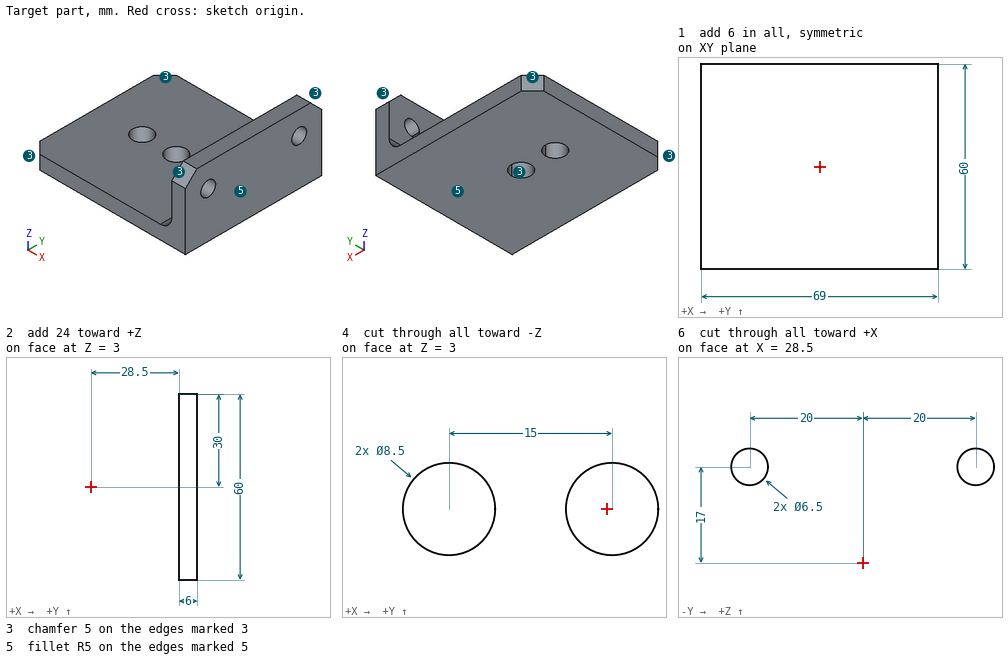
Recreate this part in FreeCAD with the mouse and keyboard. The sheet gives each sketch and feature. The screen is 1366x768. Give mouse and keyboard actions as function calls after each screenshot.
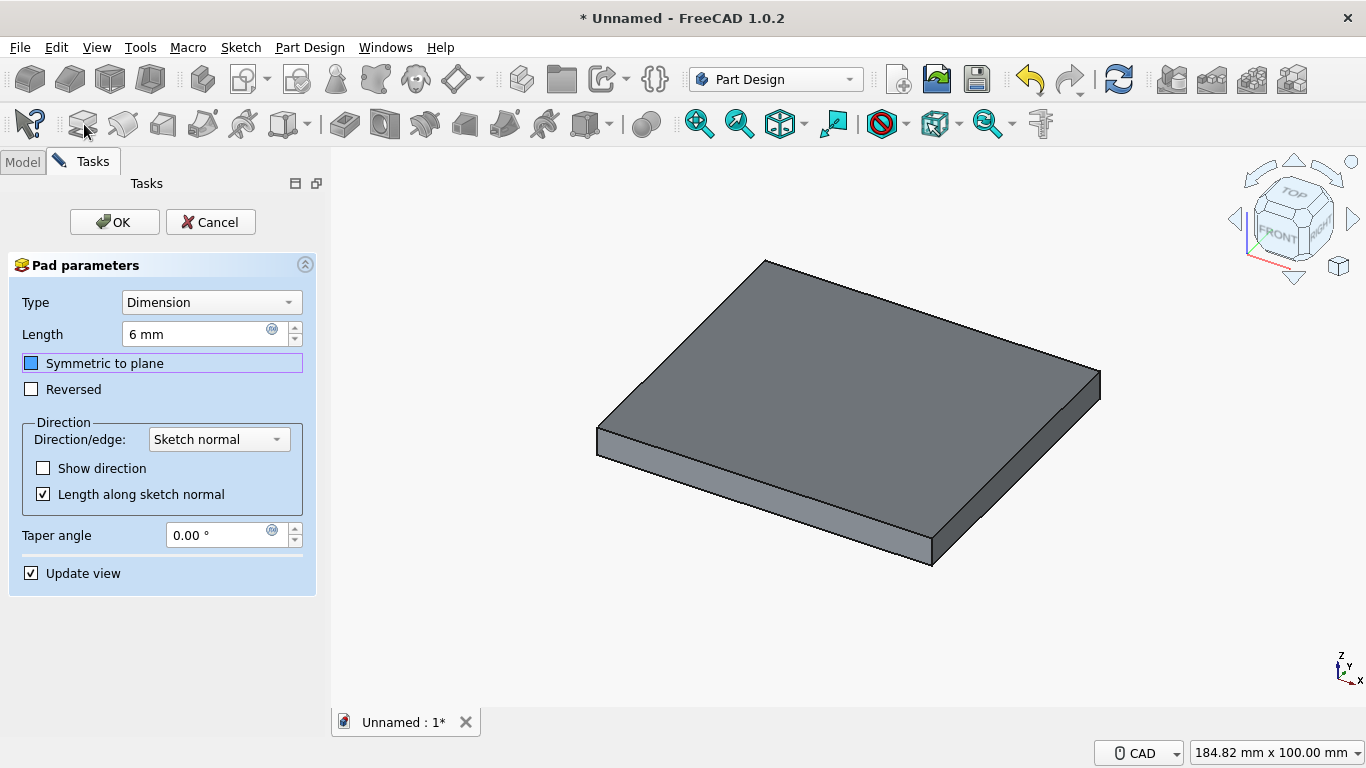
click(30, 363)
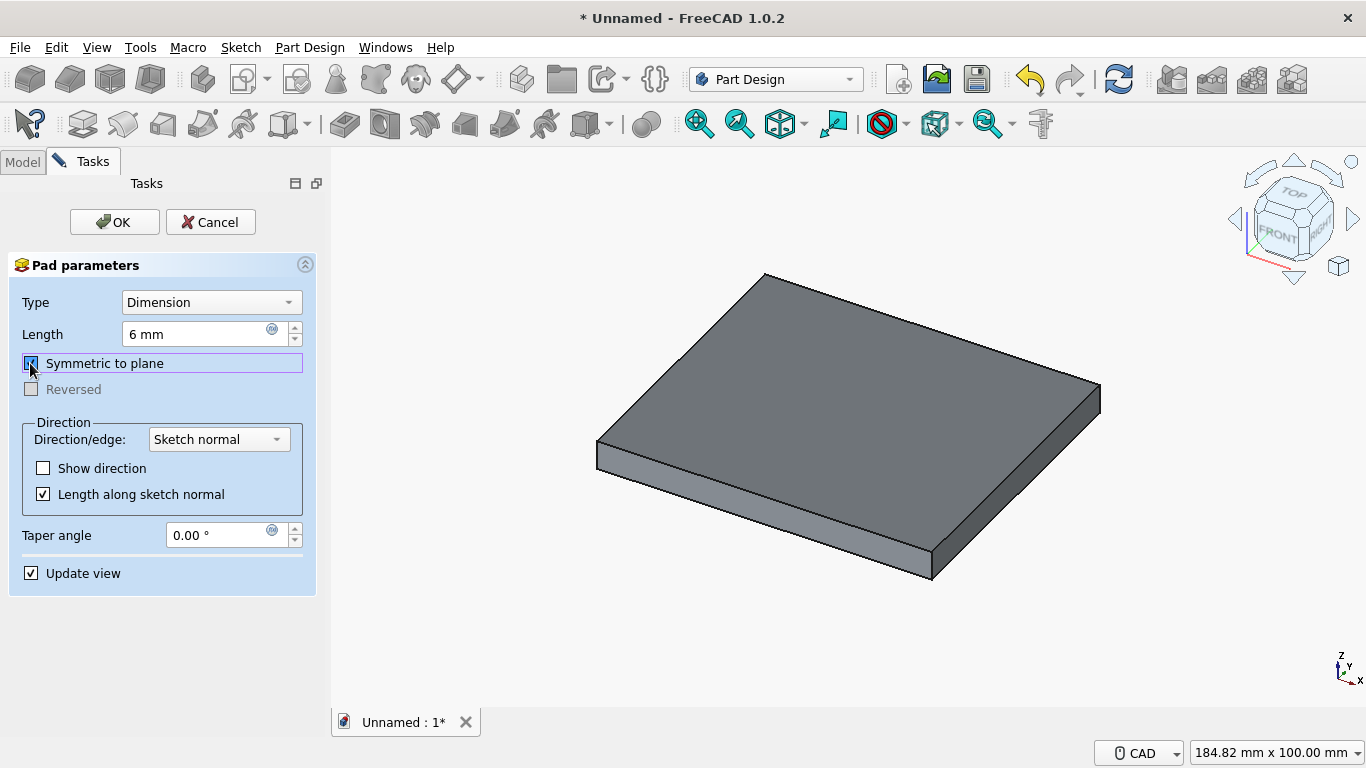
click(115, 222)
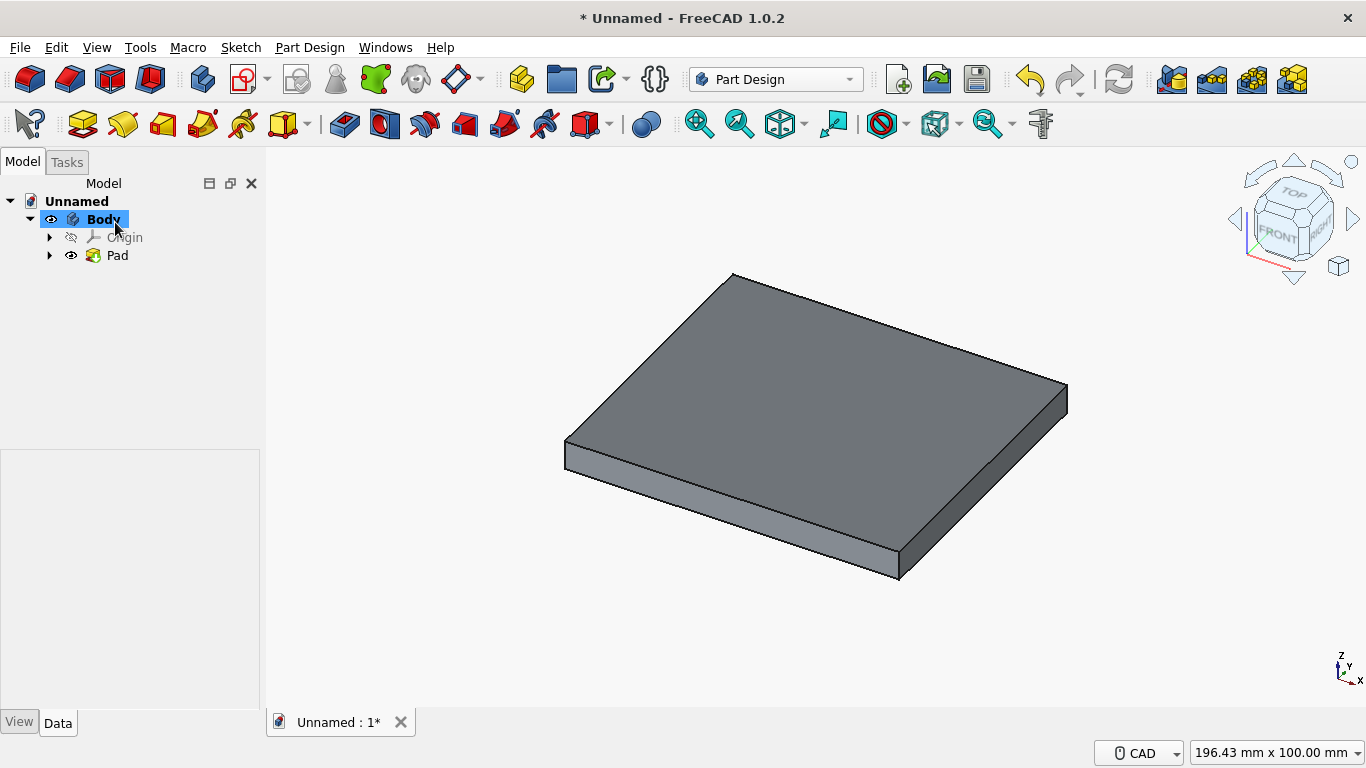
click(816, 412)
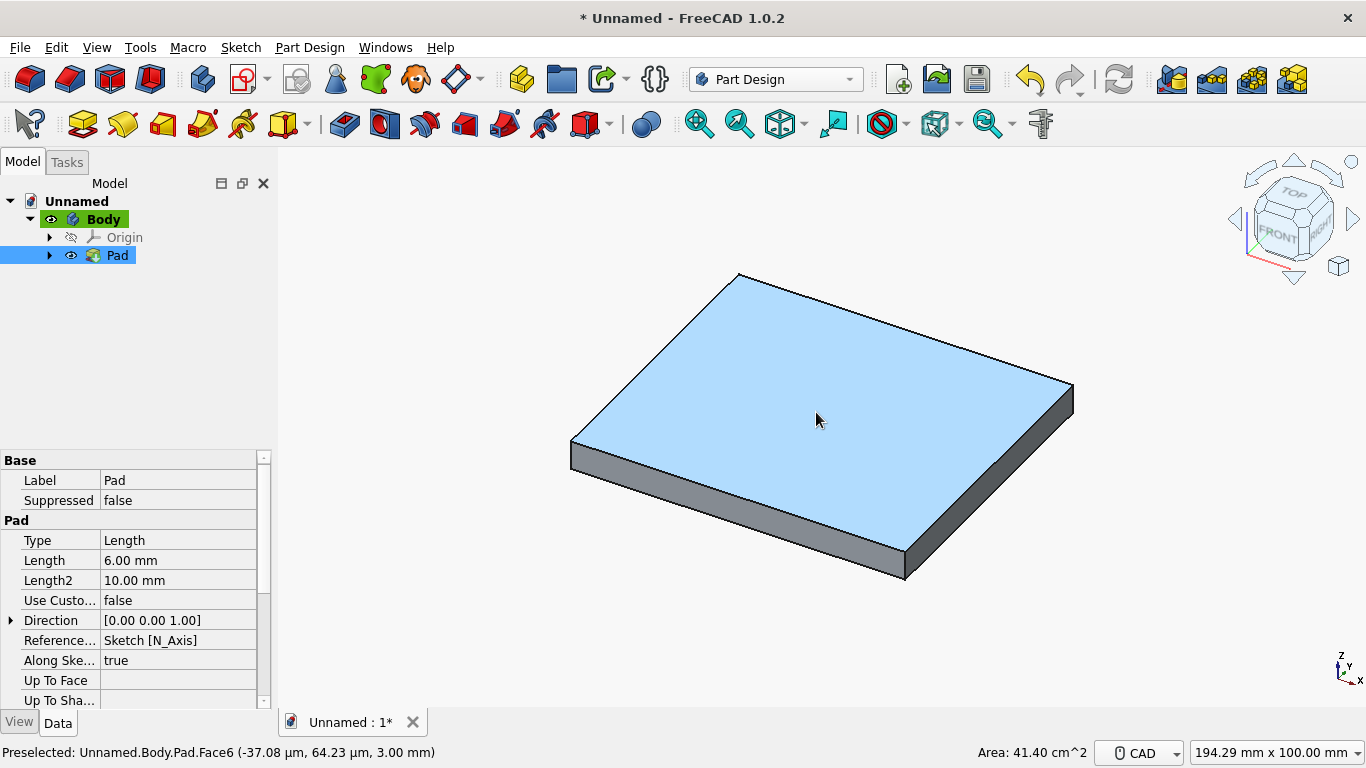
click(244, 80)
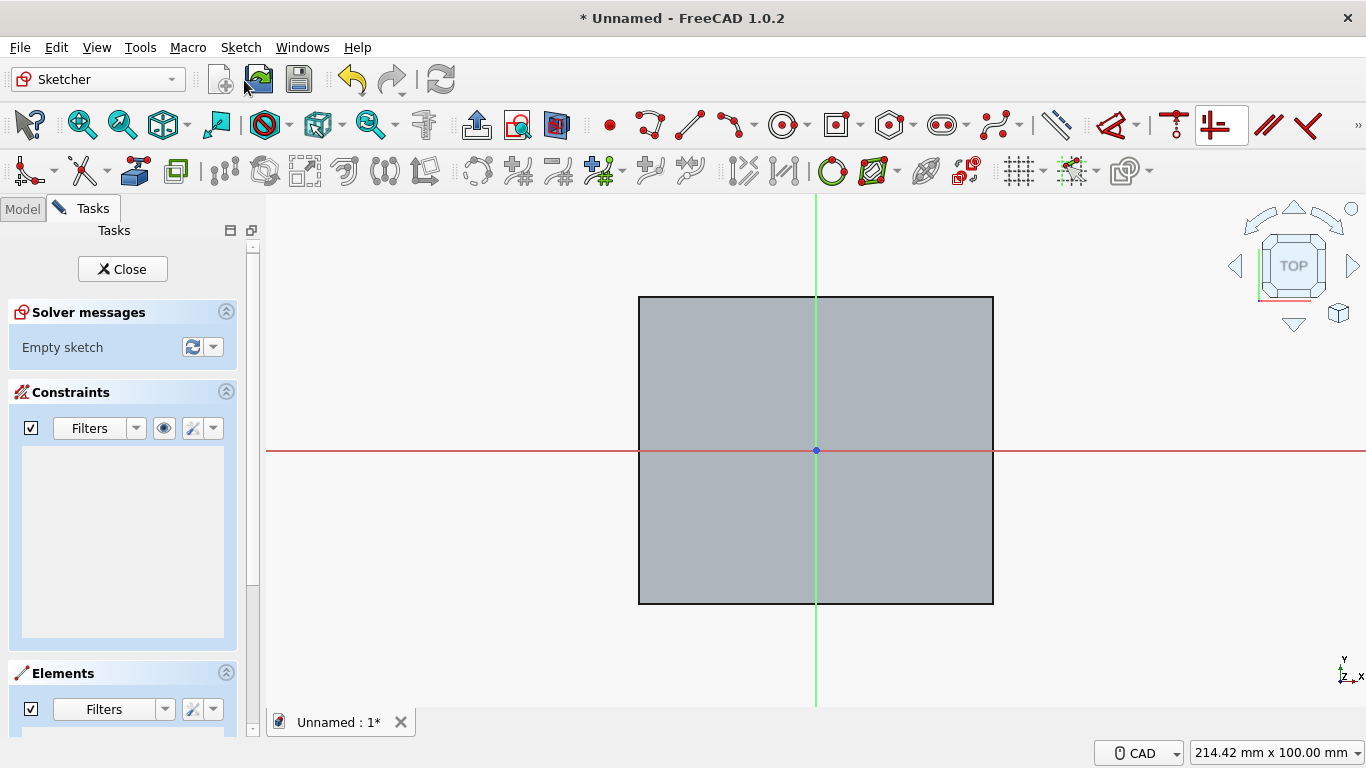
key(g)
key(r)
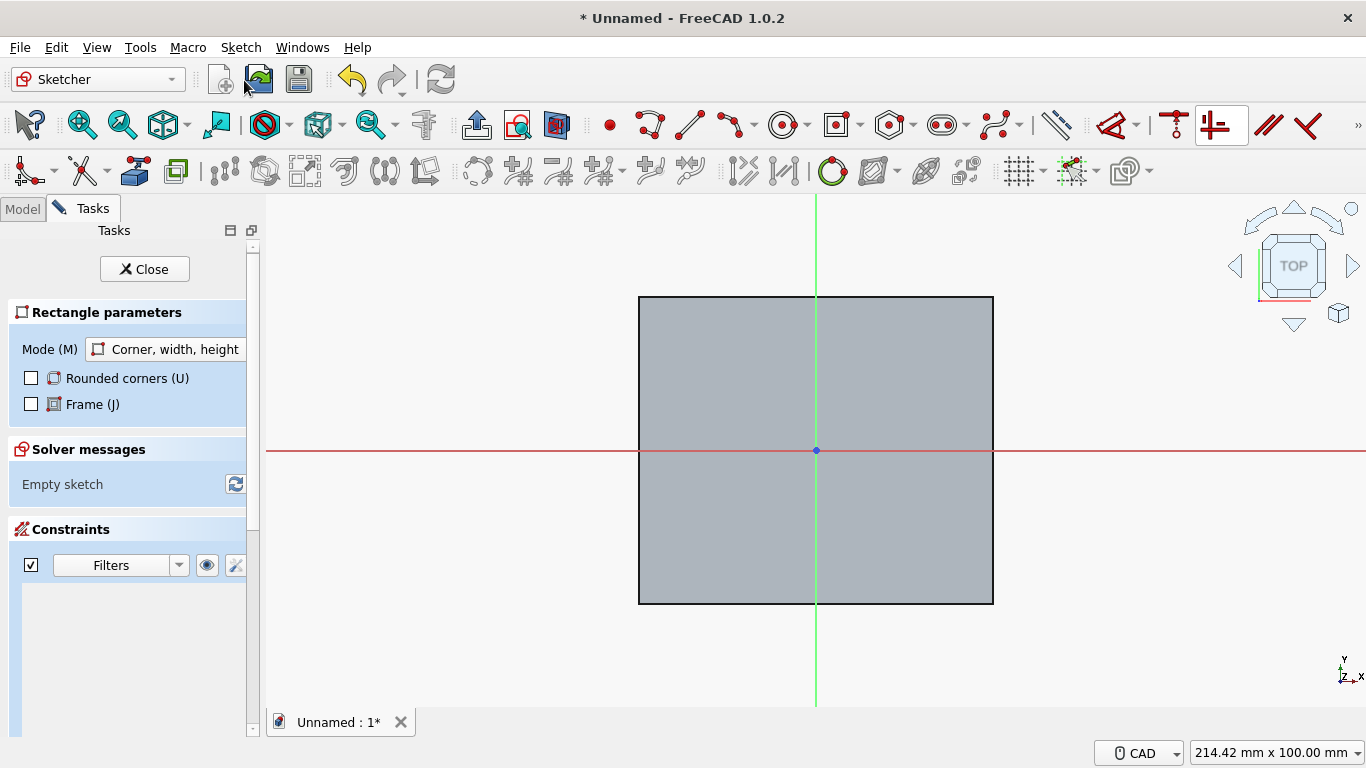
click(962, 297)
move(993, 604)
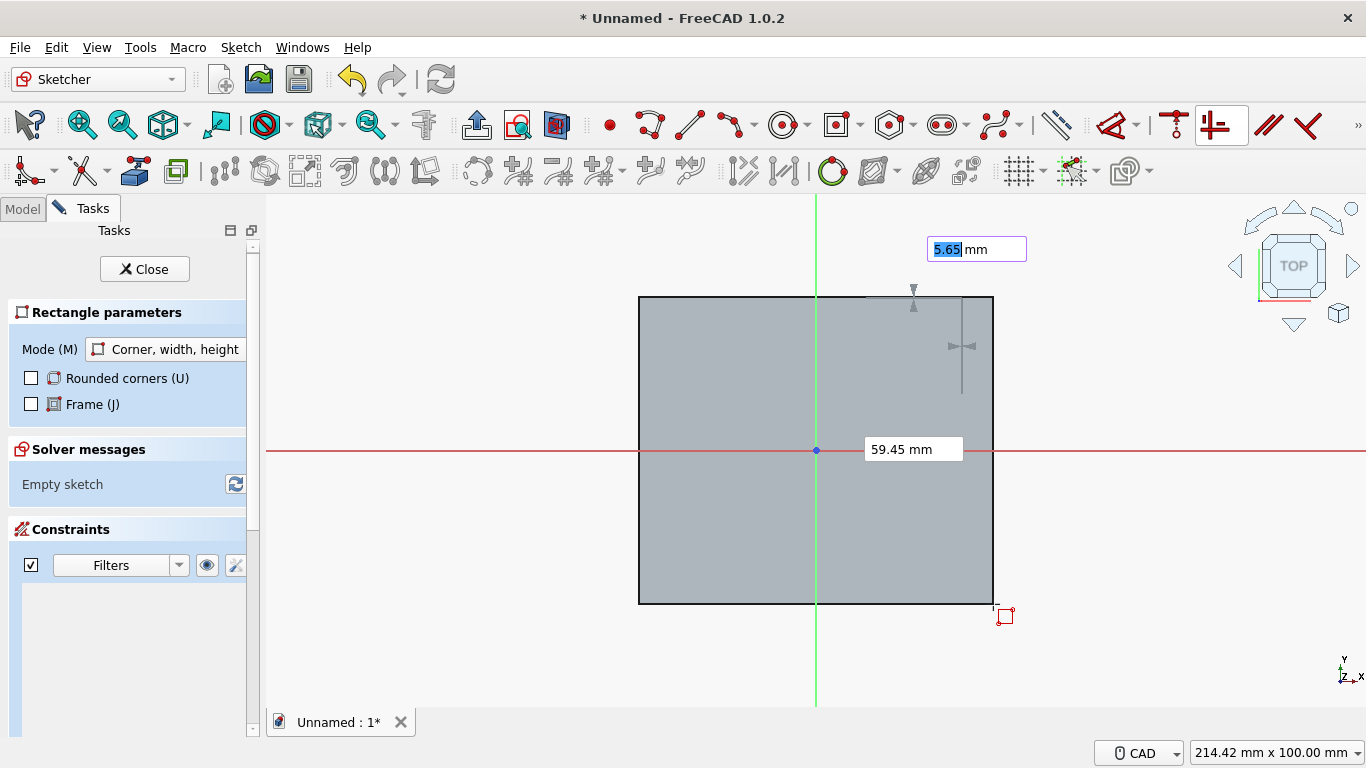
text(6)
key(Tab)
text(60)
key(Return)
key(Escape)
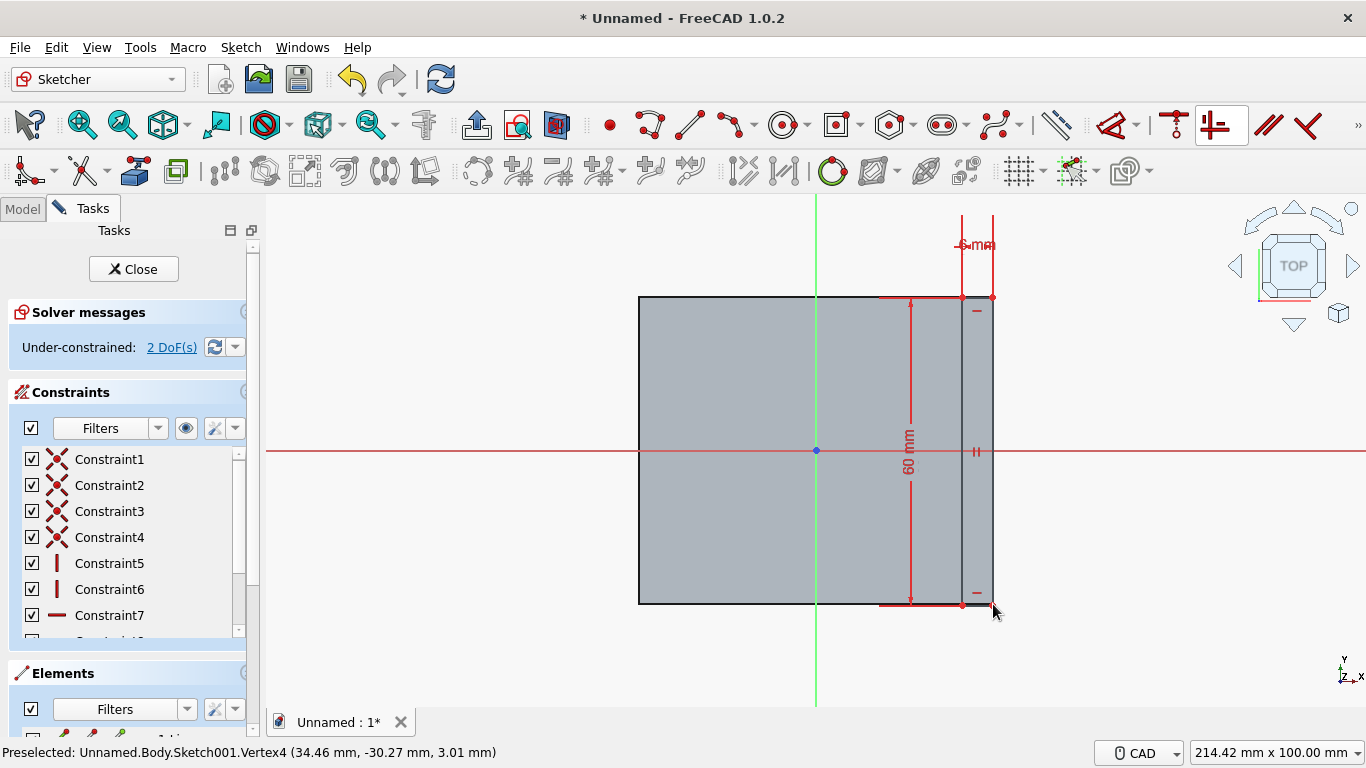
click(962, 298)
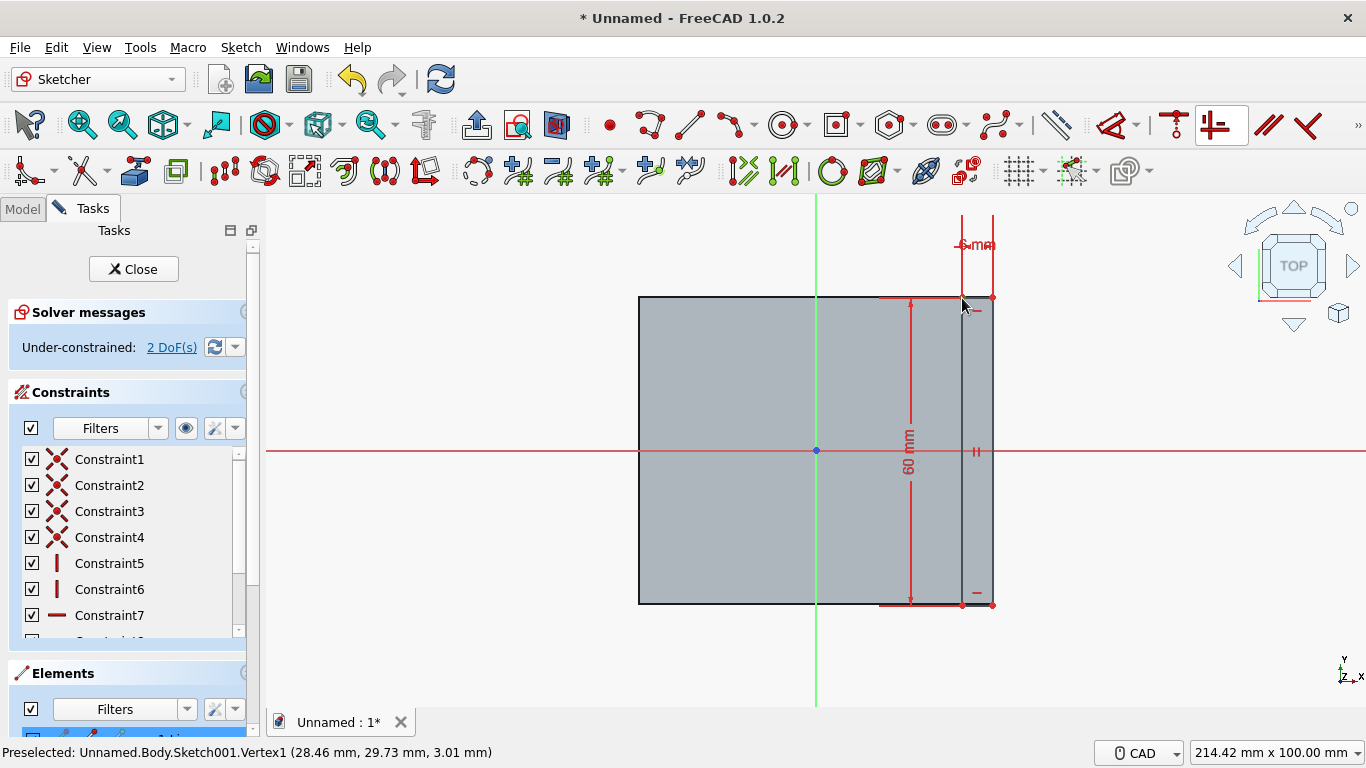
key(i)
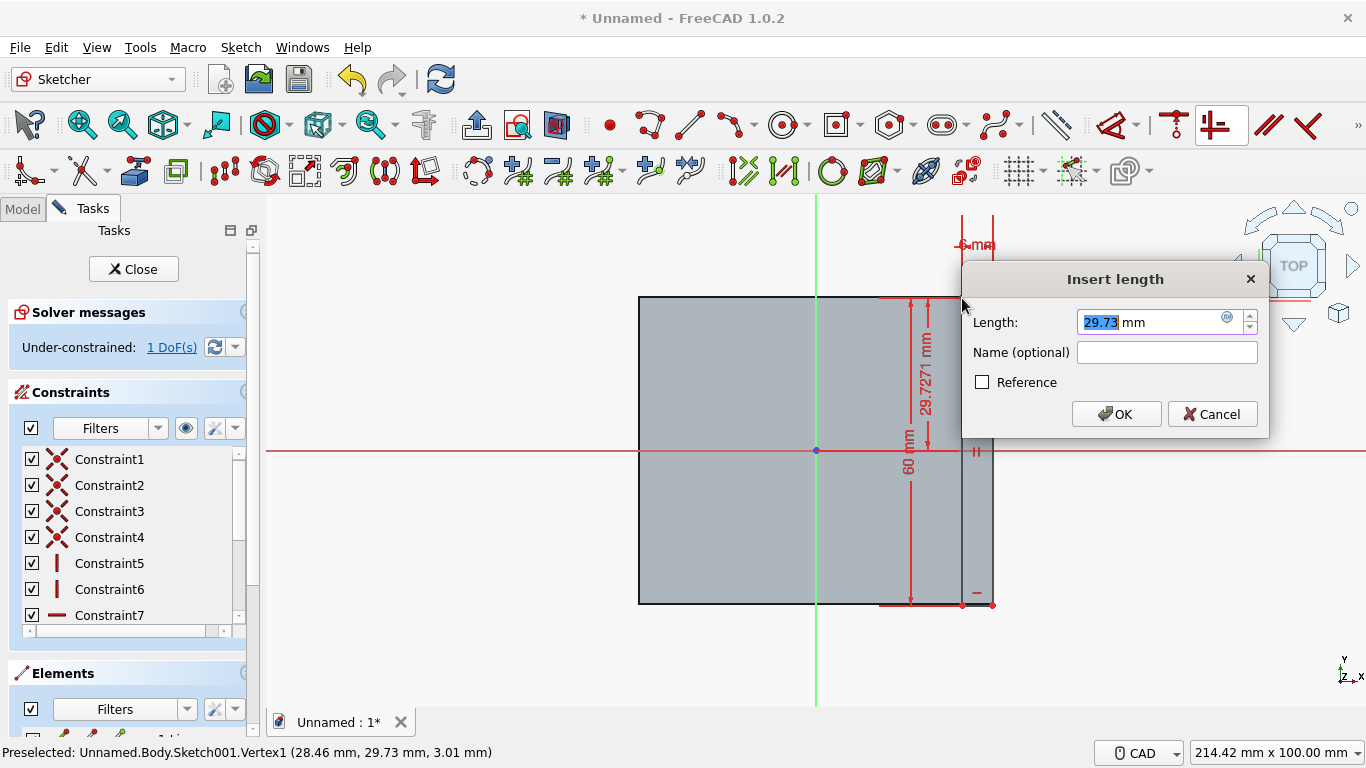
text(30)
key(Return)